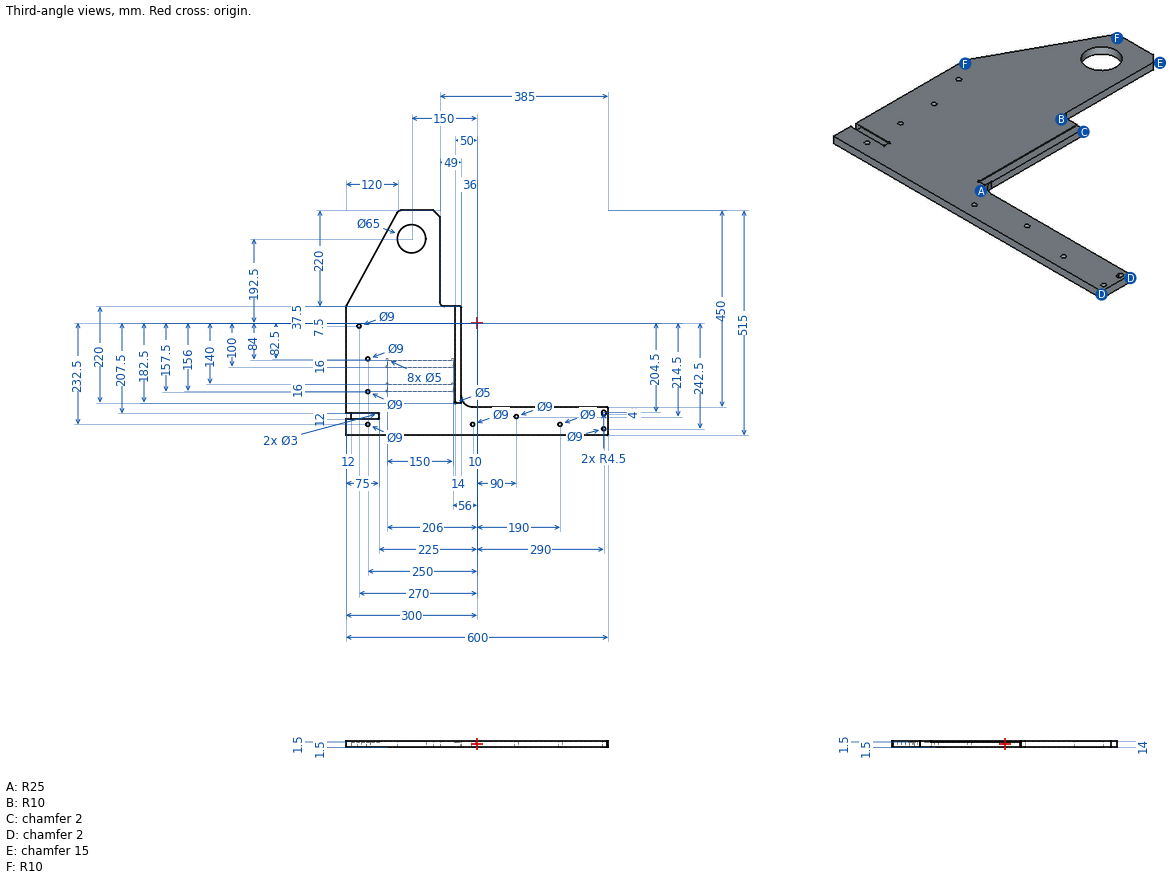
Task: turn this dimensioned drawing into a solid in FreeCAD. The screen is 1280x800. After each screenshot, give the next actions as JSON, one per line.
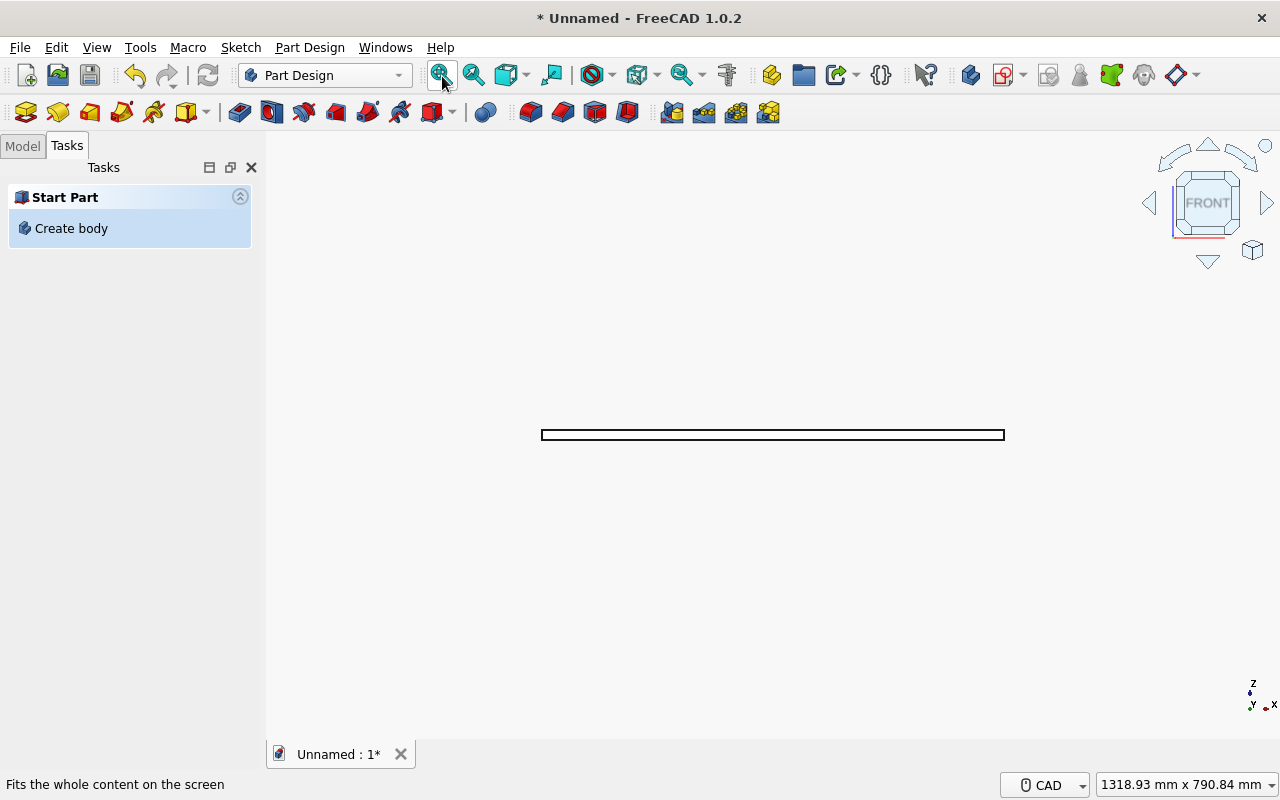
{"action": "scroll", "coordinate": [708, 434], "scroll_direction": "up", "scroll_amount": 7}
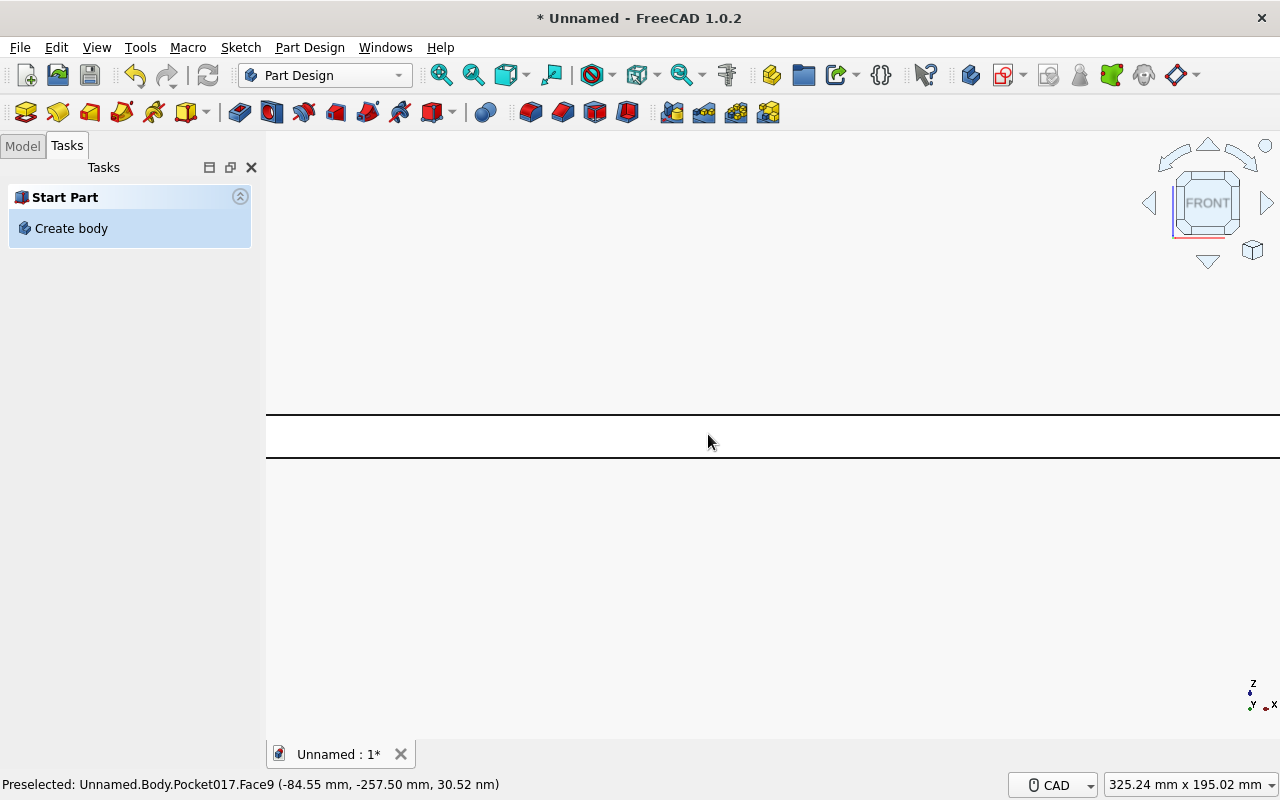
{"action": "left_click", "coordinate": [442, 76]}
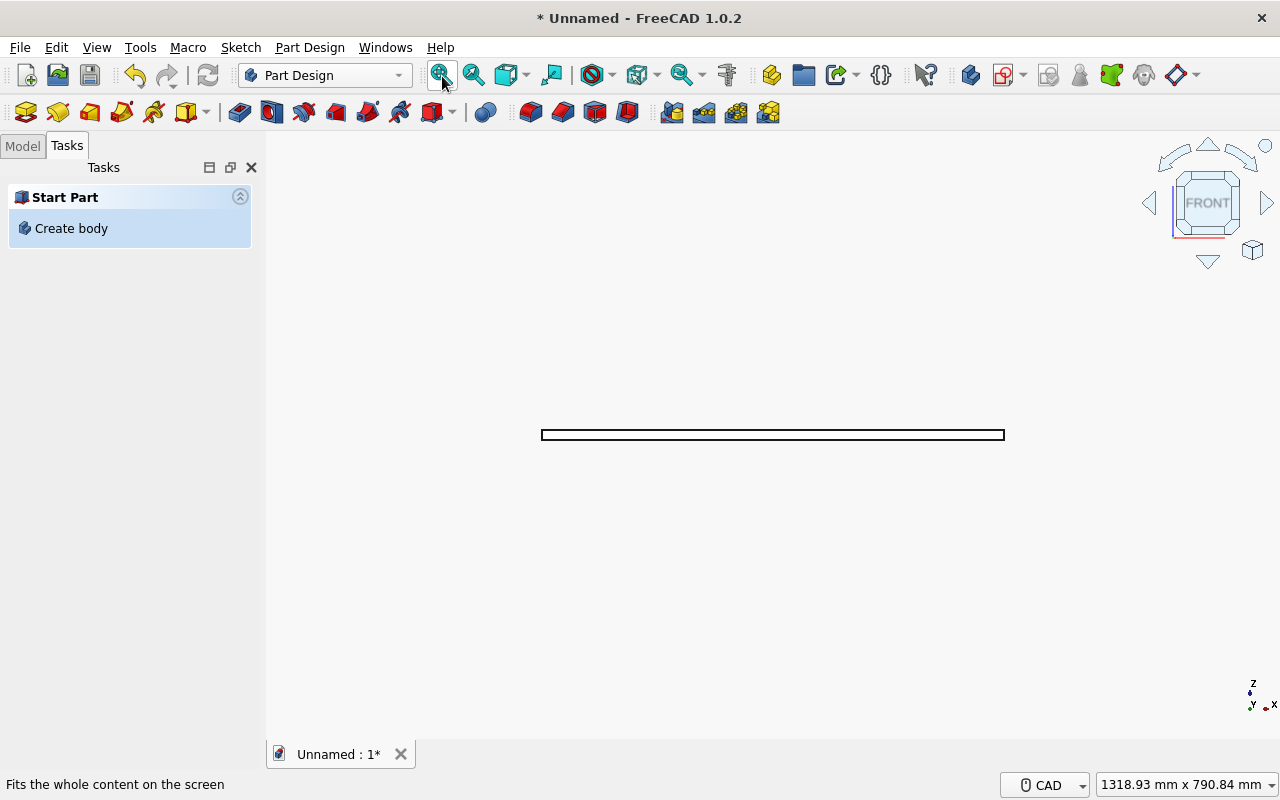
{"action": "key", "text": "3"}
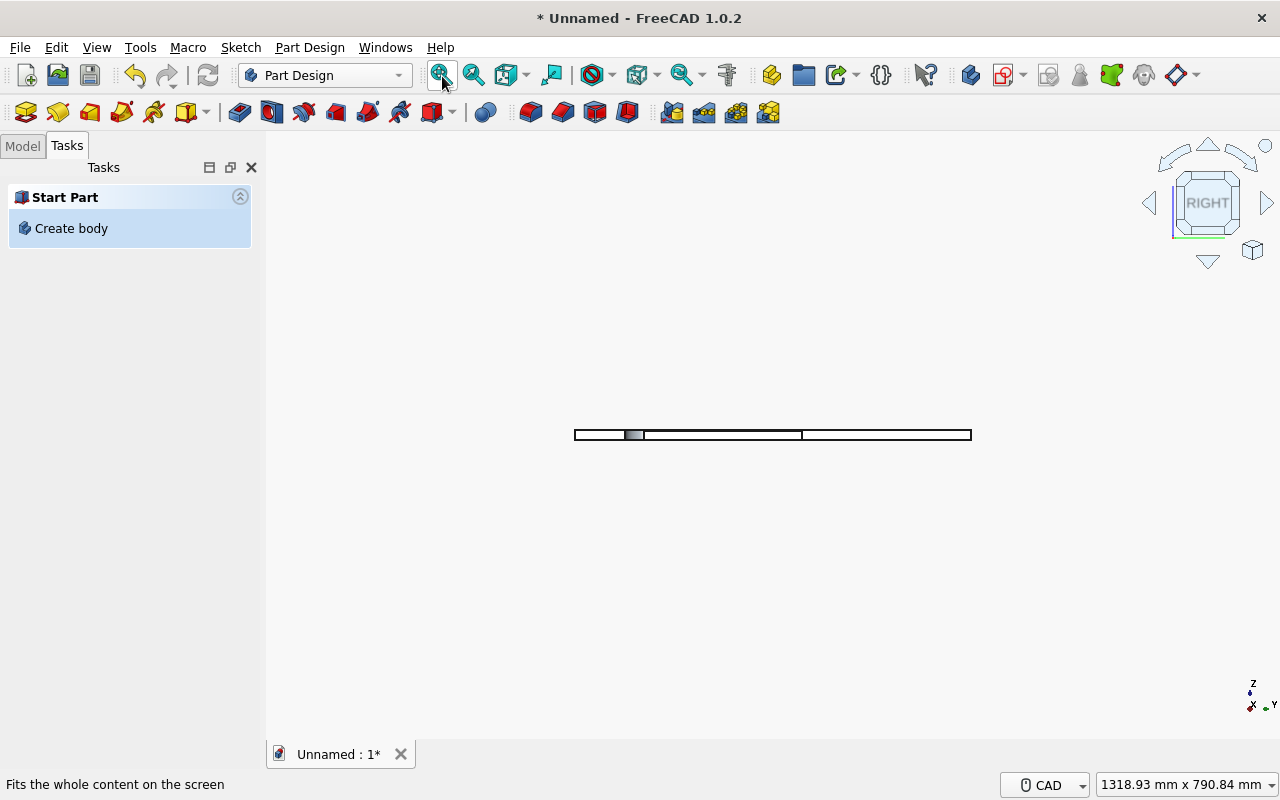
{"action": "left_click", "coordinate": [442, 76]}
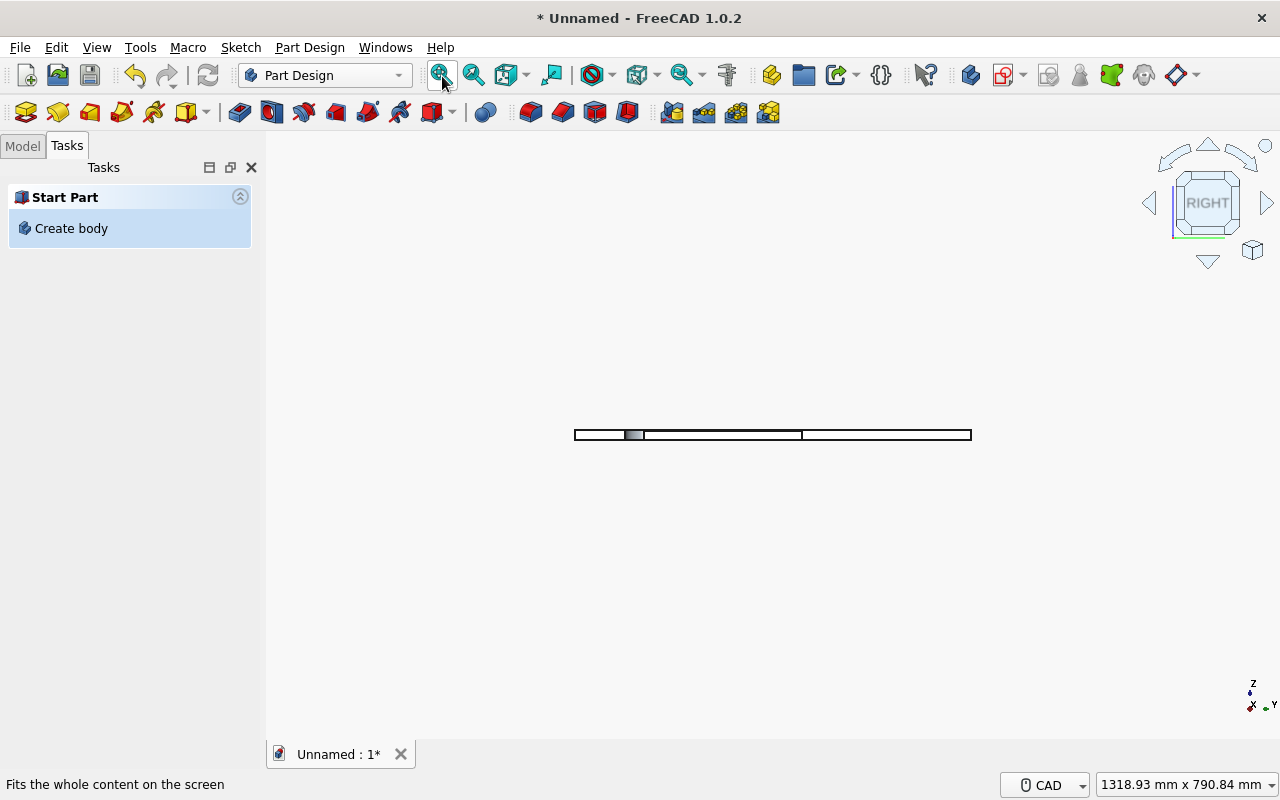
{"action": "scroll", "coordinate": [802, 434], "scroll_direction": "up", "scroll_amount": 7}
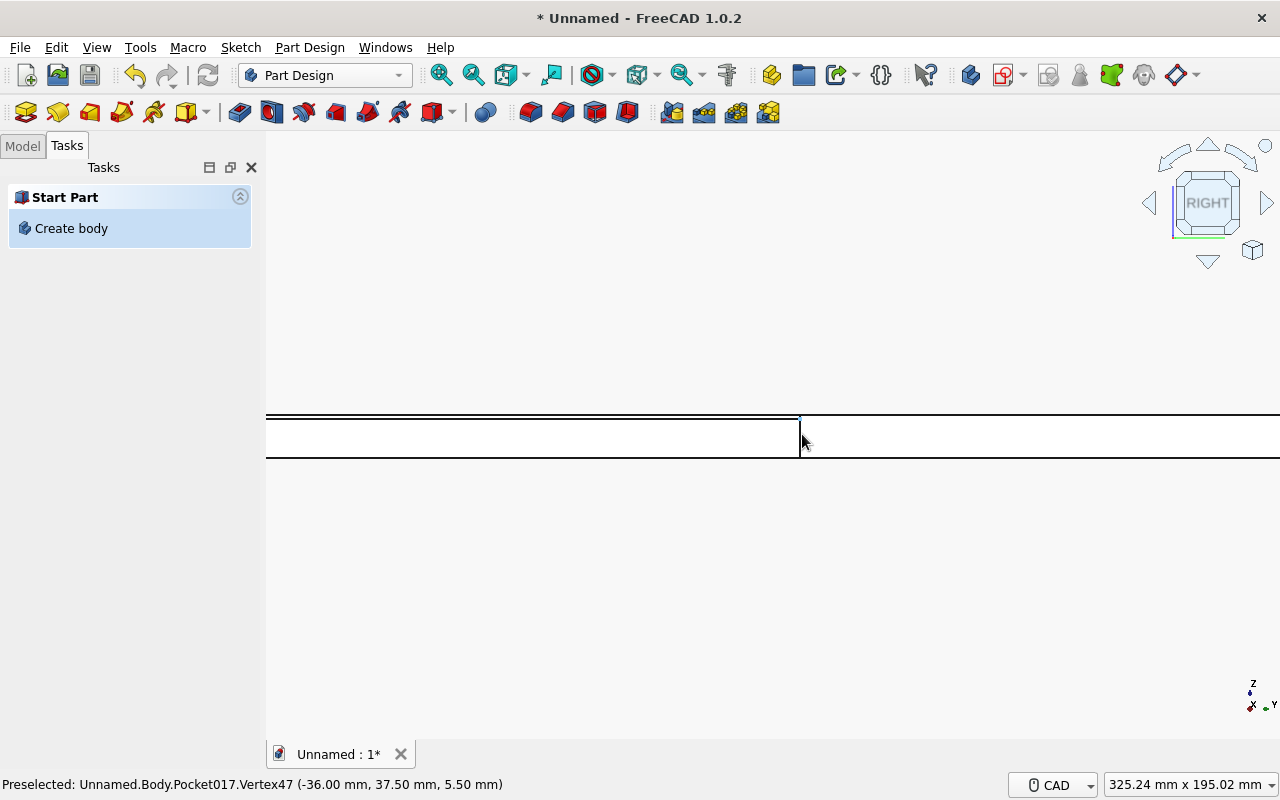
{"action": "left_click", "coordinate": [442, 76]}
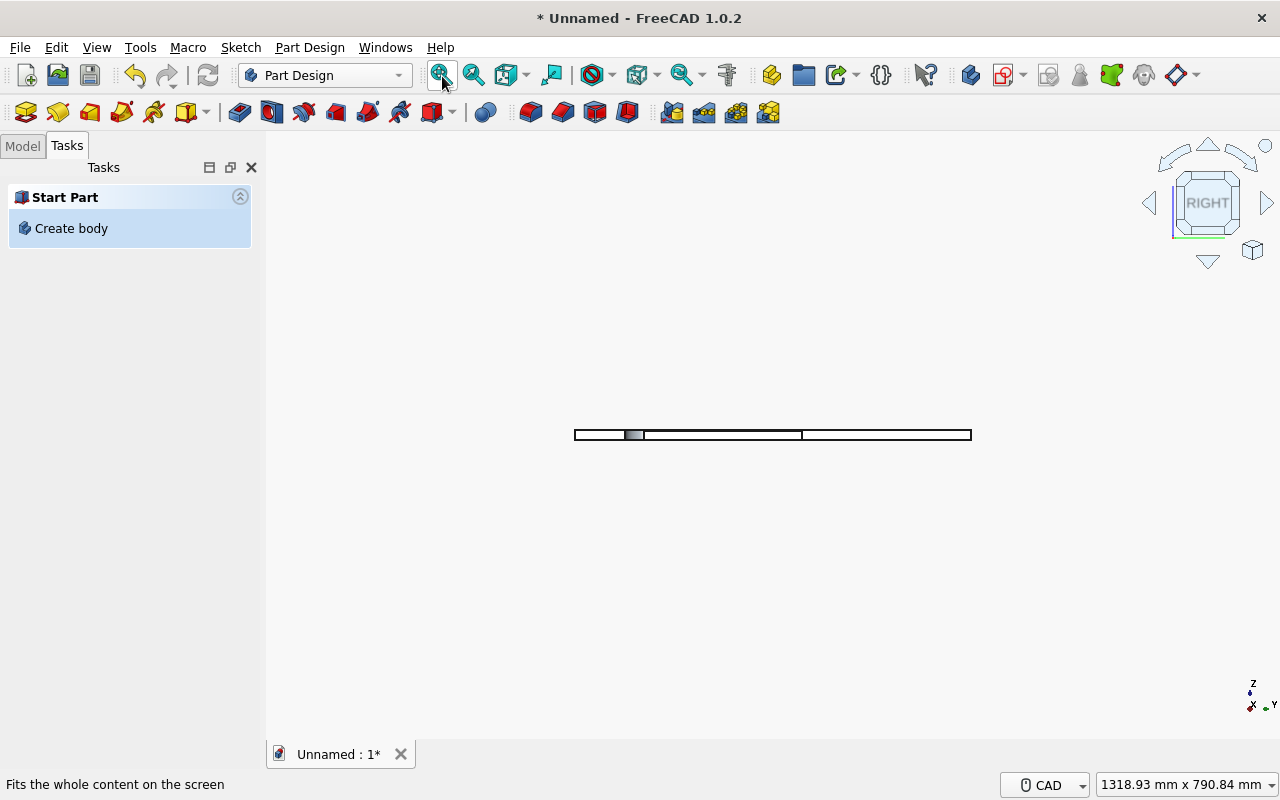
{"action": "key", "text": "5"}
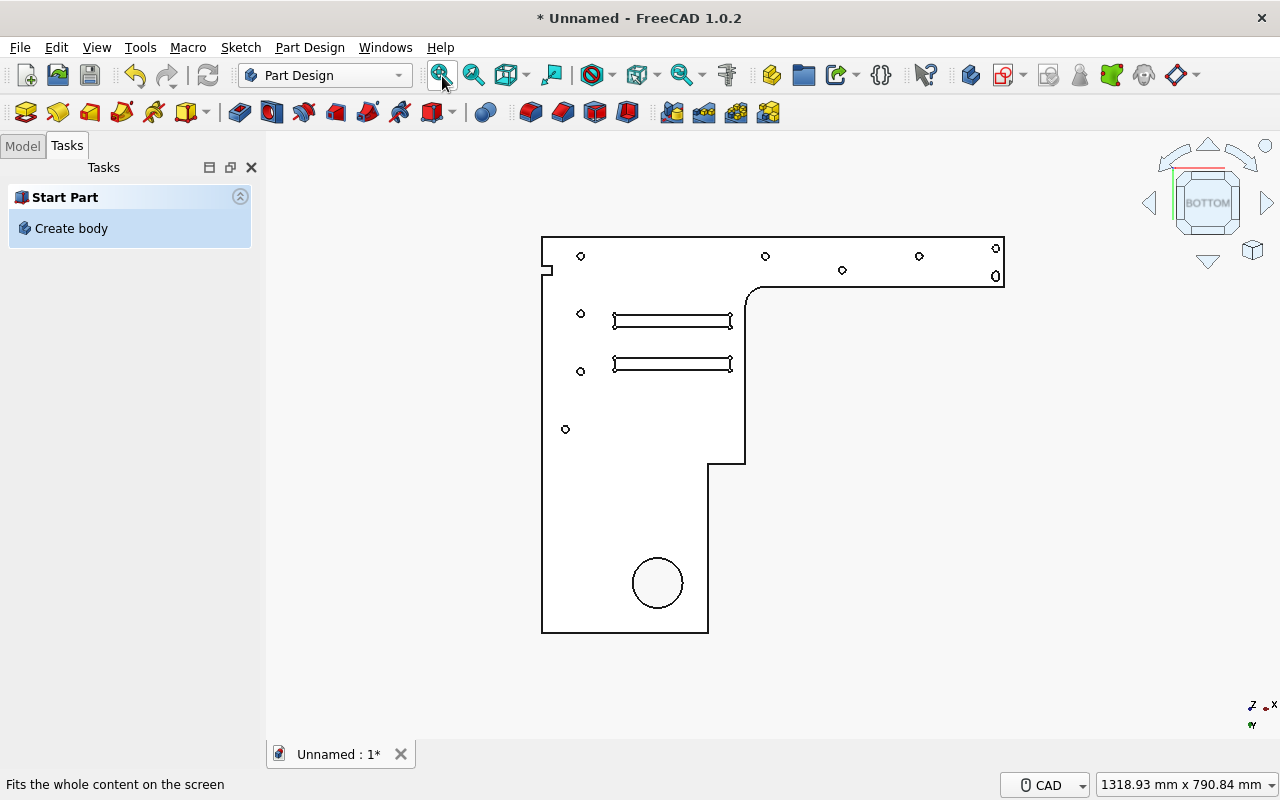
{"action": "scroll", "coordinate": [708, 463], "scroll_direction": "up", "scroll_amount": 7}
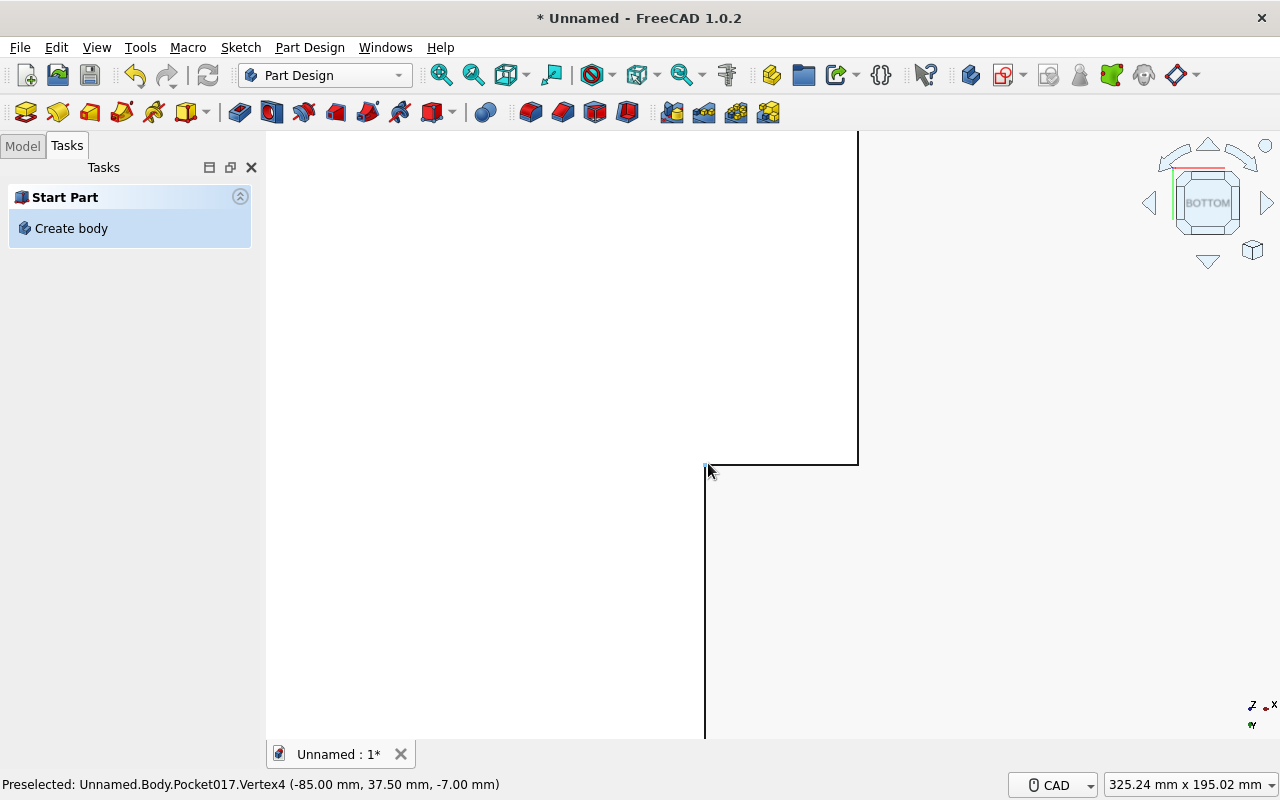
{"action": "left_click", "coordinate": [442, 76]}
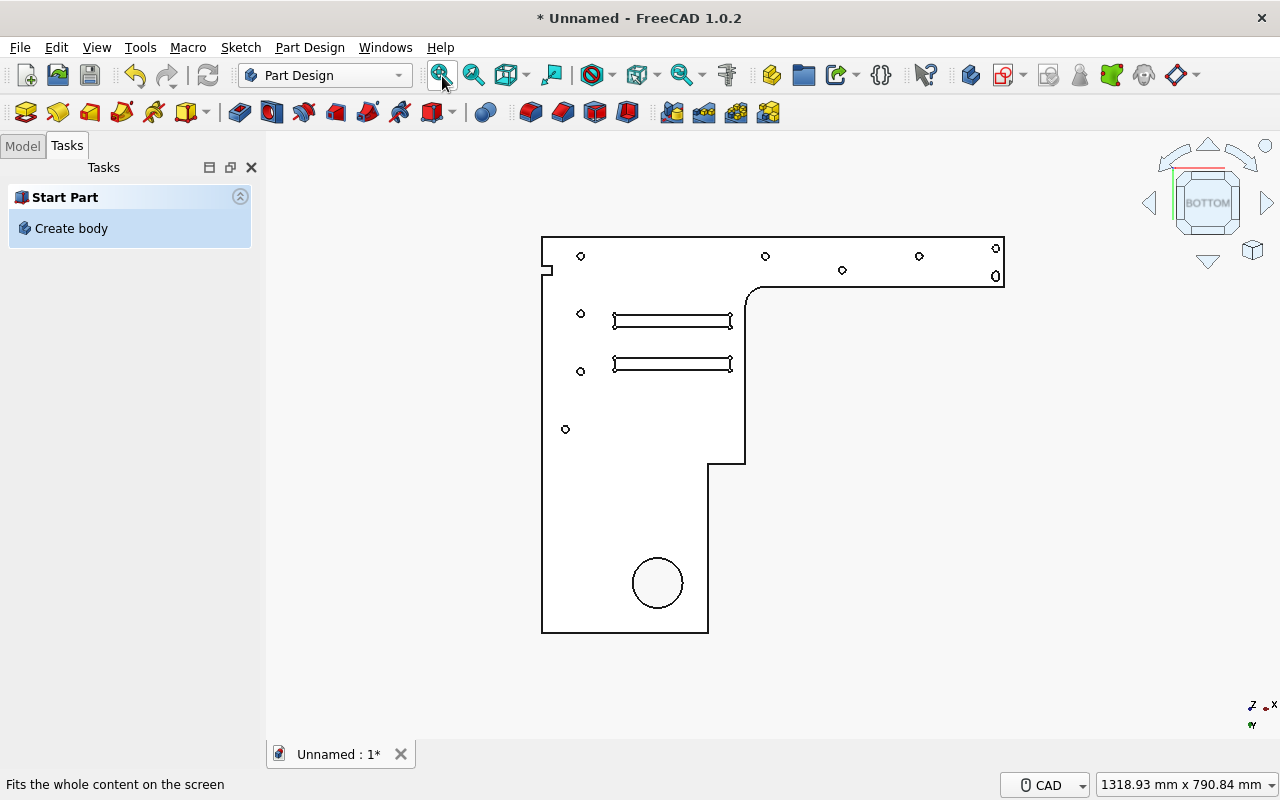
{"action": "key", "text": "4"}